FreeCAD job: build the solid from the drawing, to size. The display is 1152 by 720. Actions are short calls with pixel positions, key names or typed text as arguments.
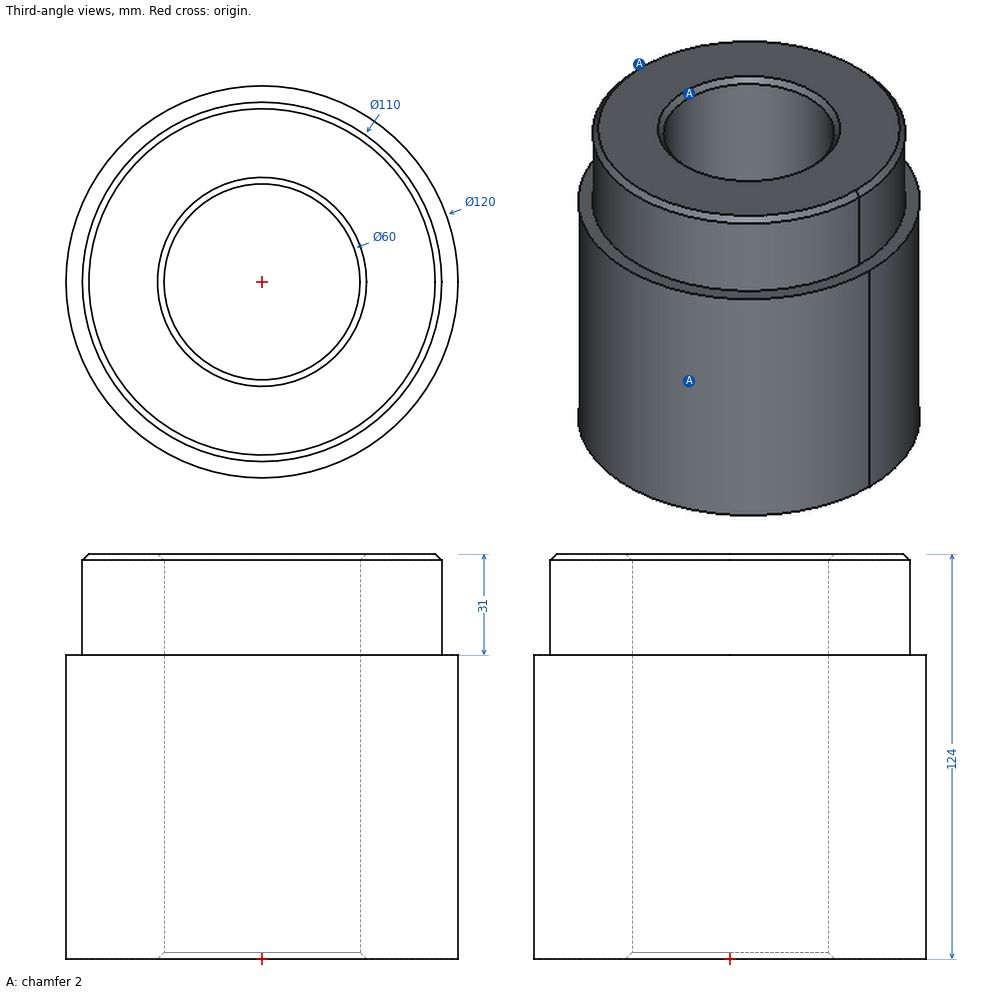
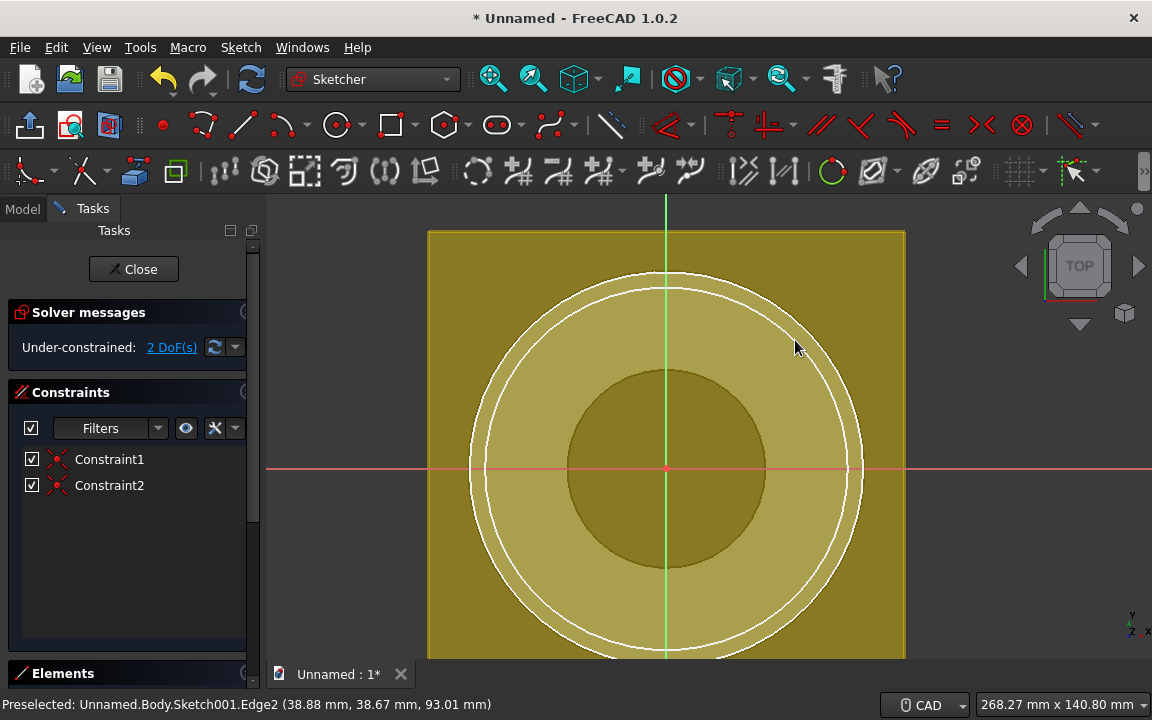
click(666, 126)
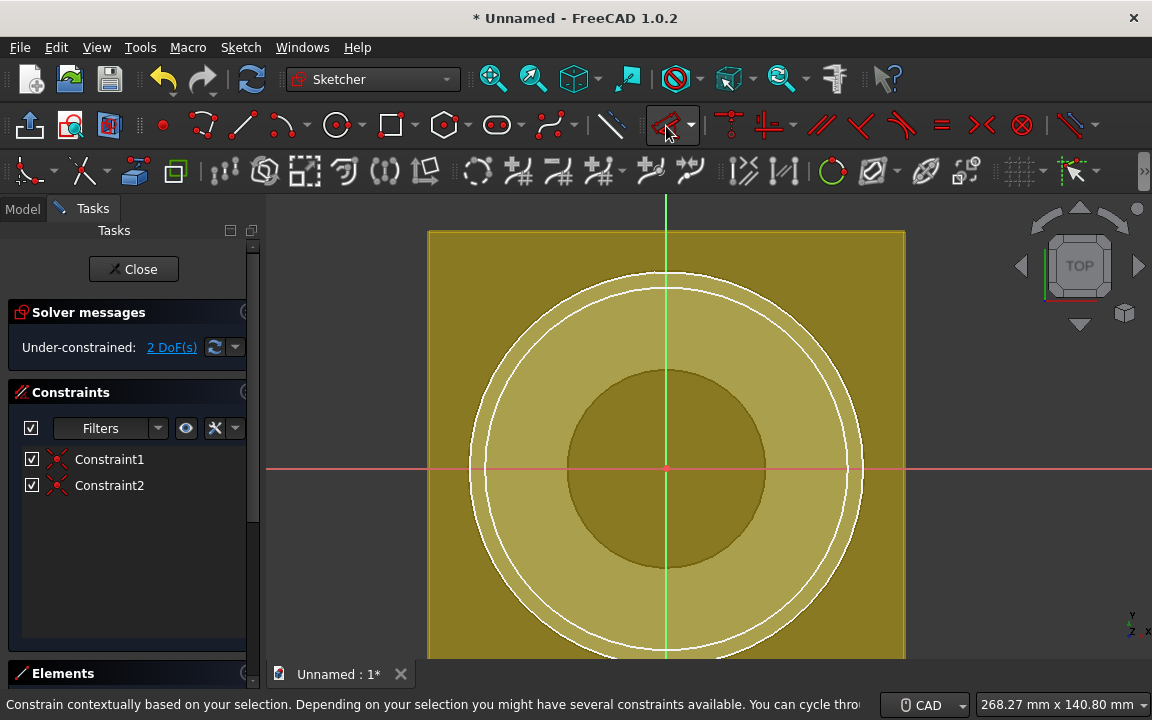
click(805, 329)
click(828, 306)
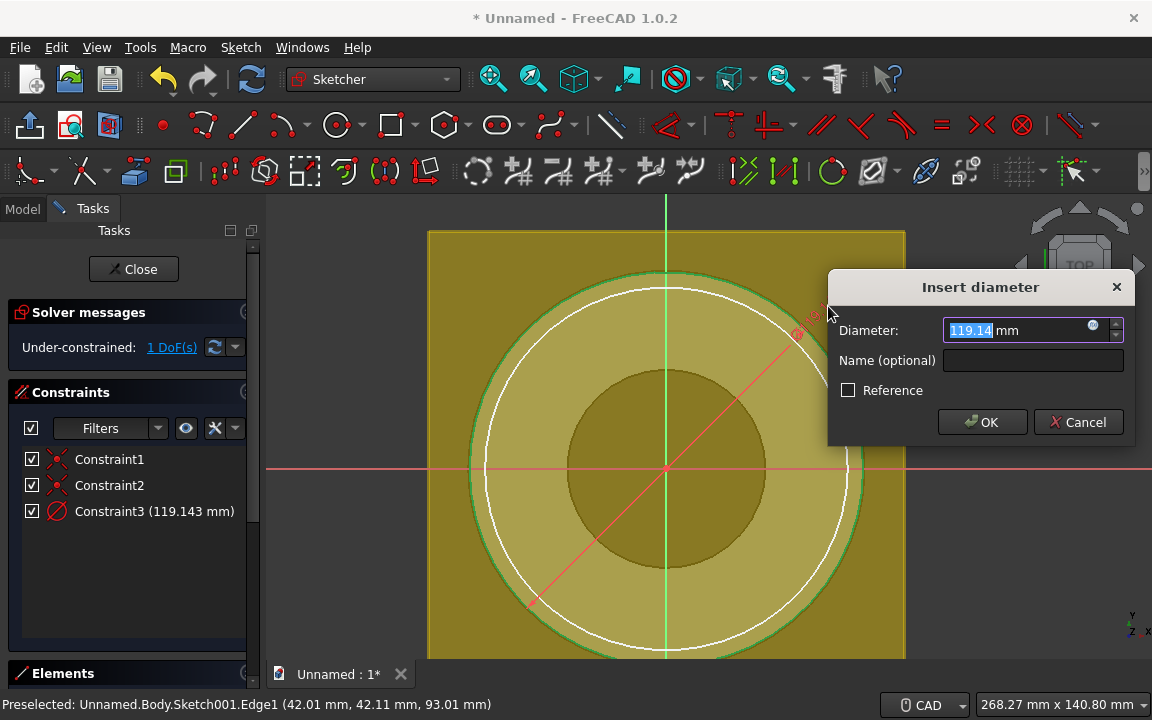
text(120)
key(Return)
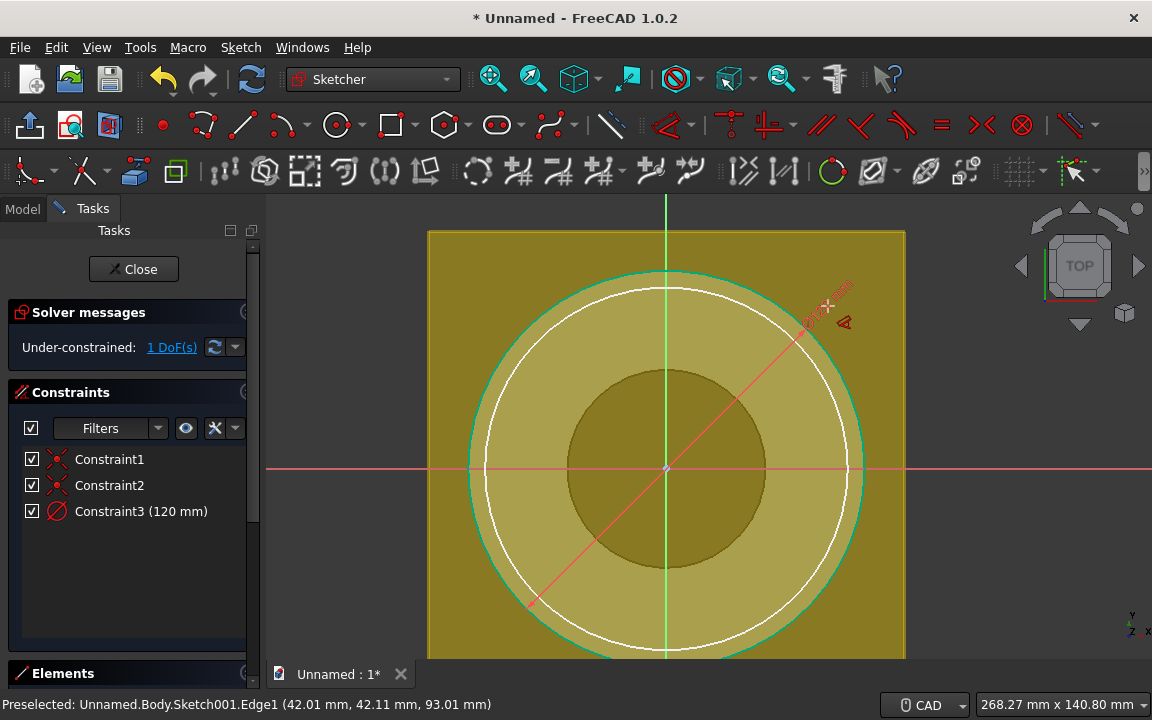
click(794, 340)
click(871, 408)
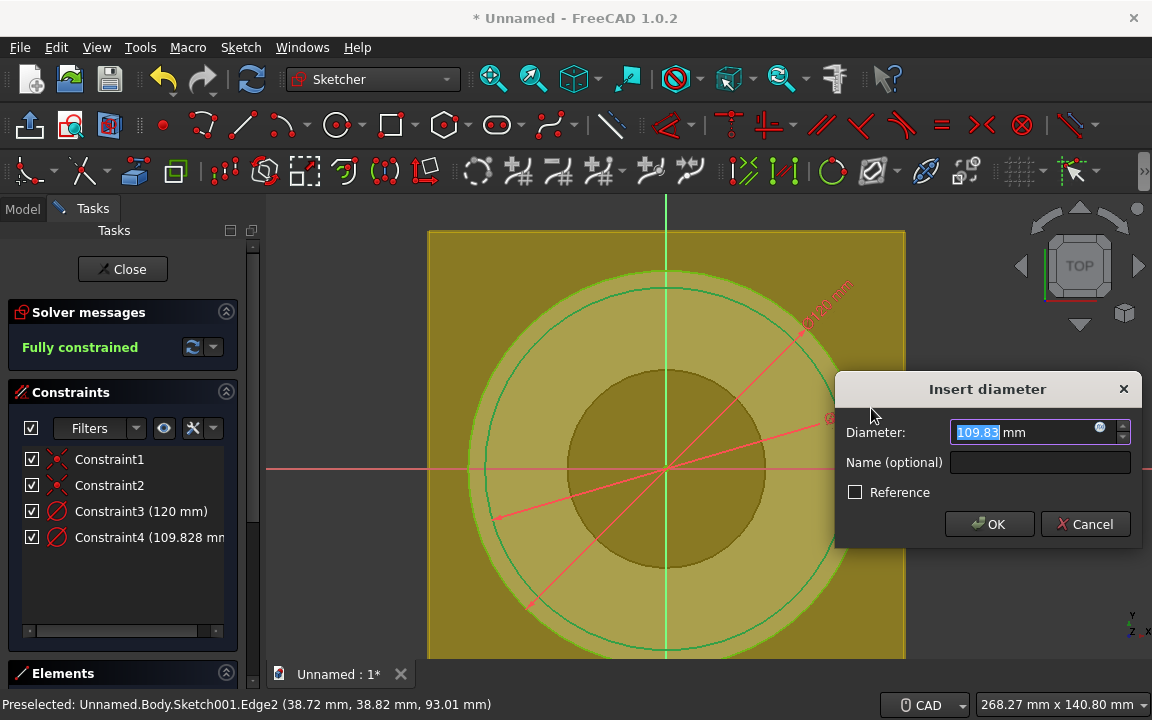
text(110)
key(Return)
key(Escape)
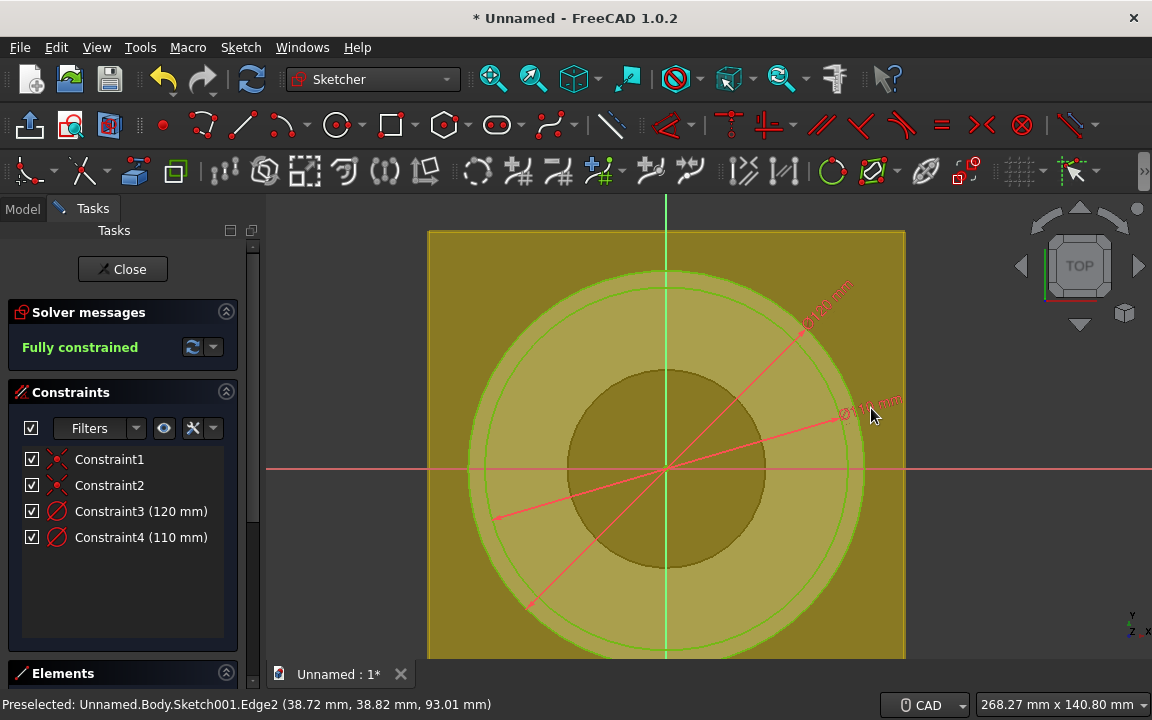
click(123, 269)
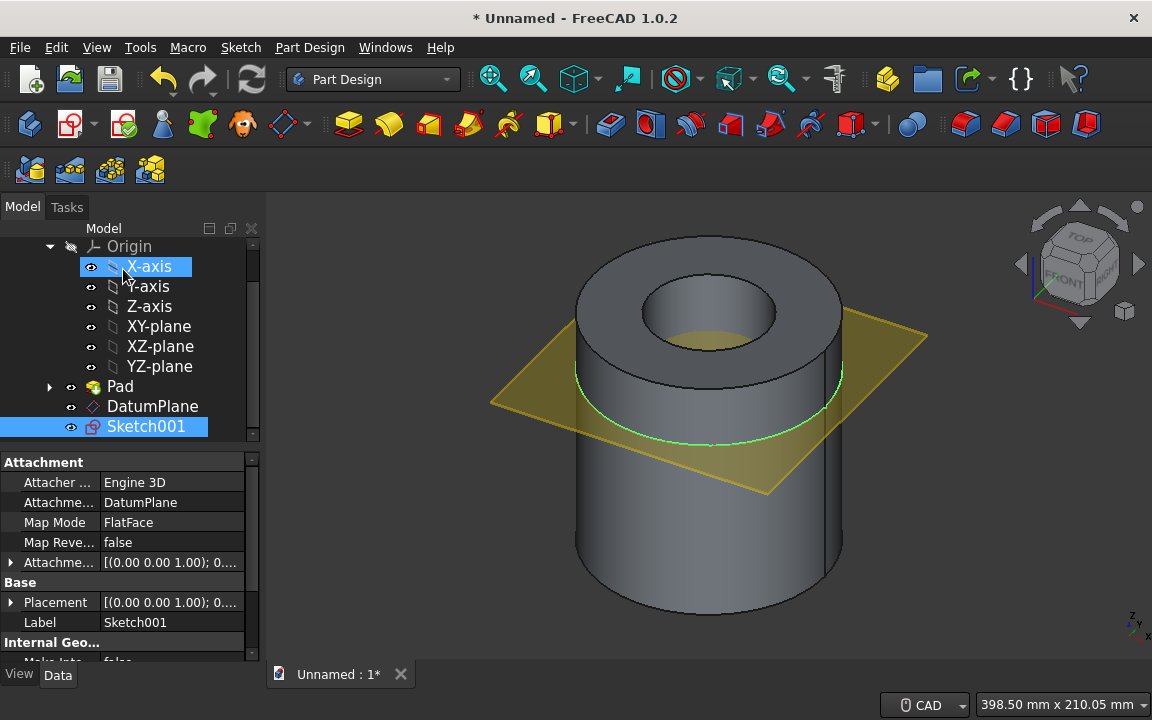
click(612, 124)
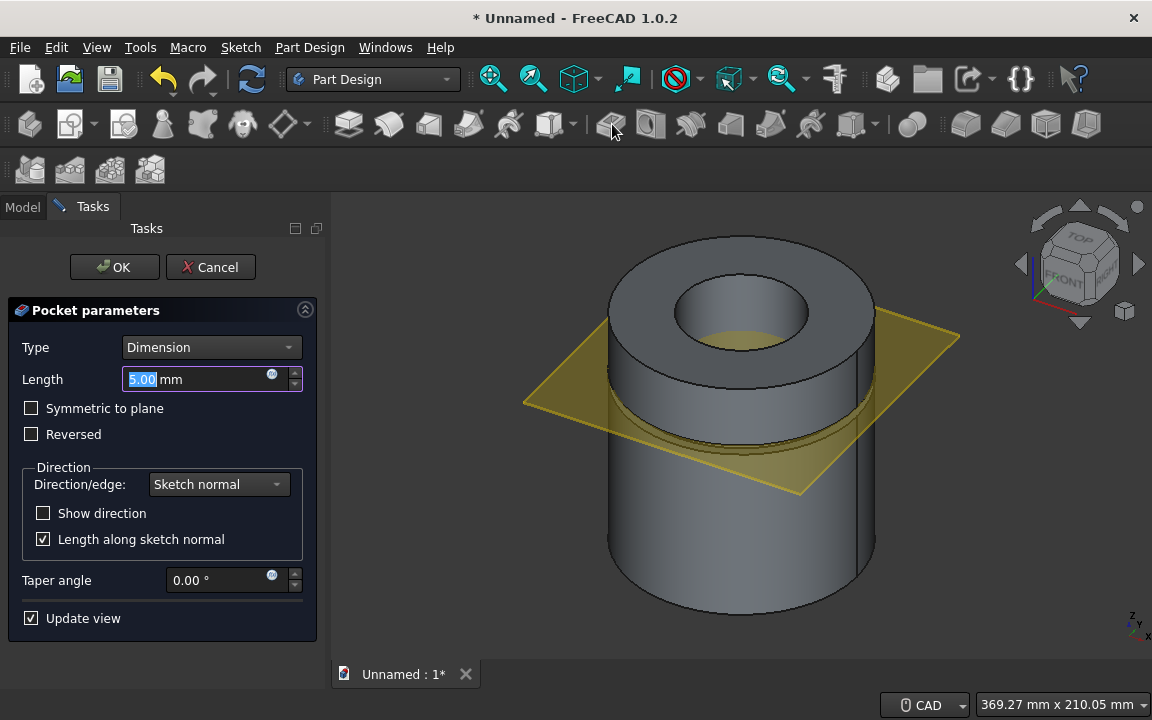
text(31)
key(Tab)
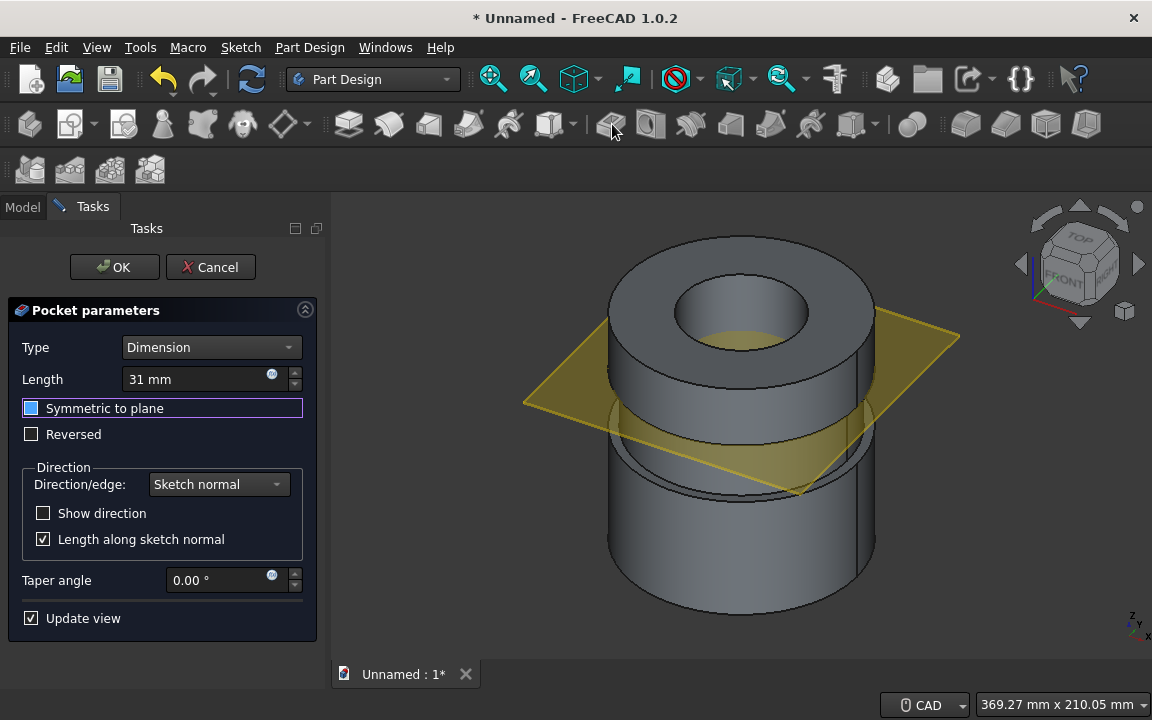
click(30, 434)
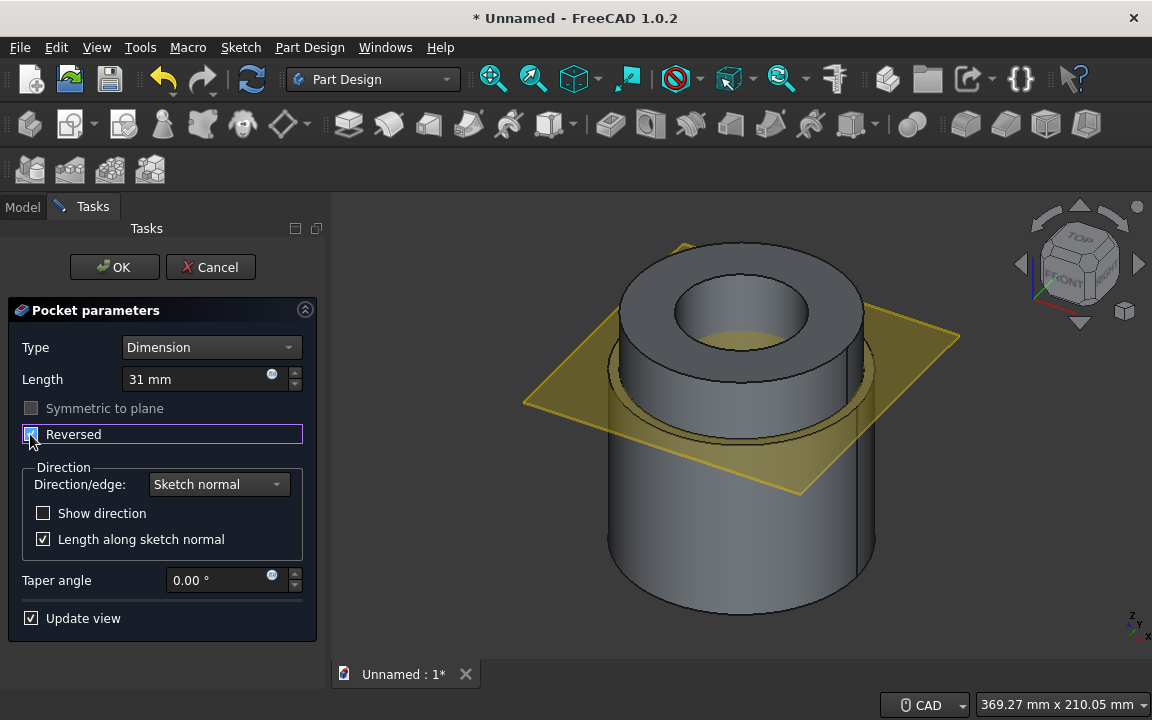
click(115, 267)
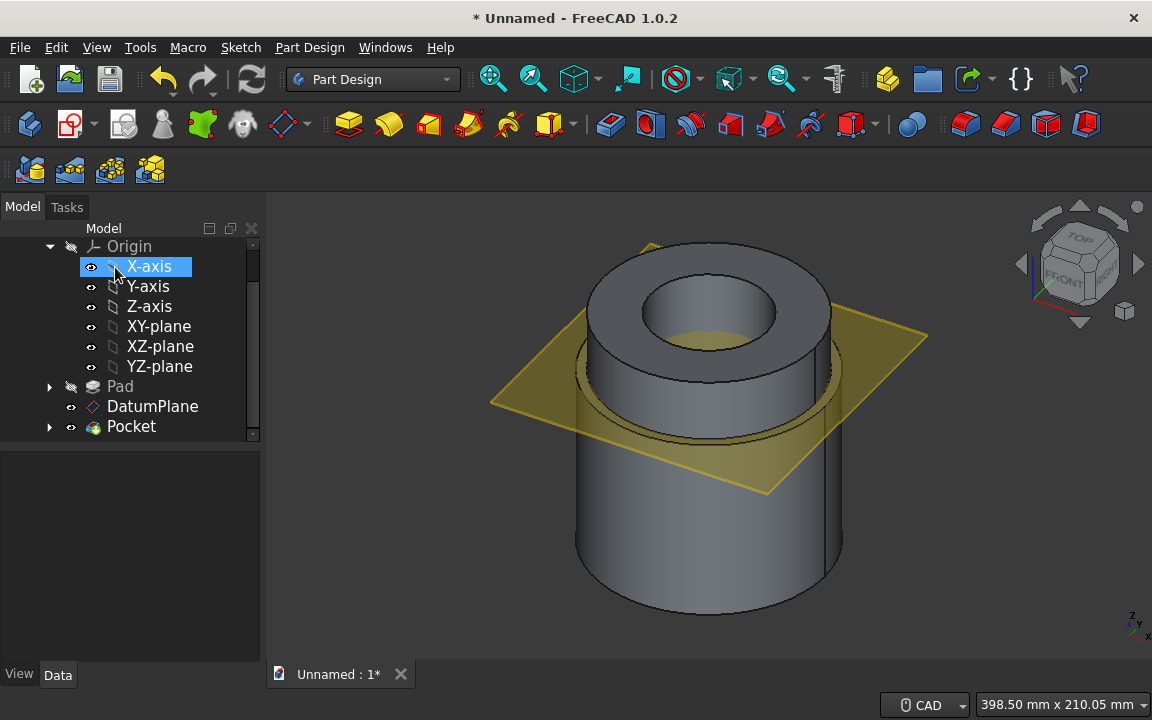
click(116, 407)
key(space)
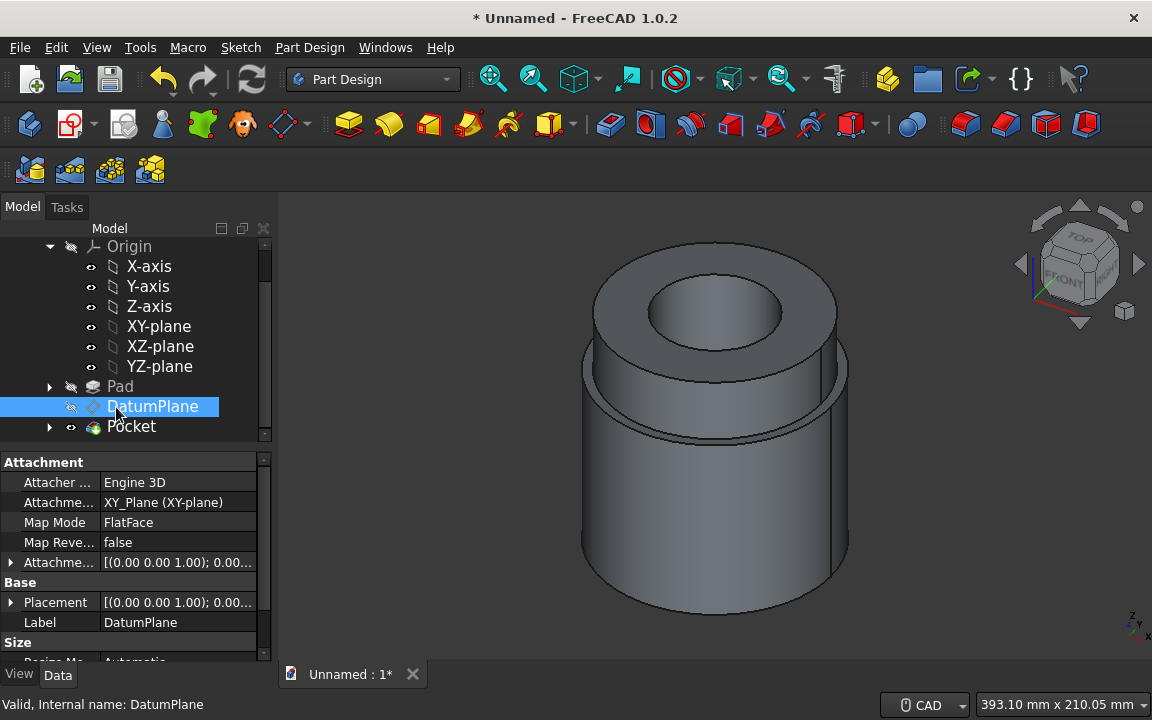
click(593, 319)